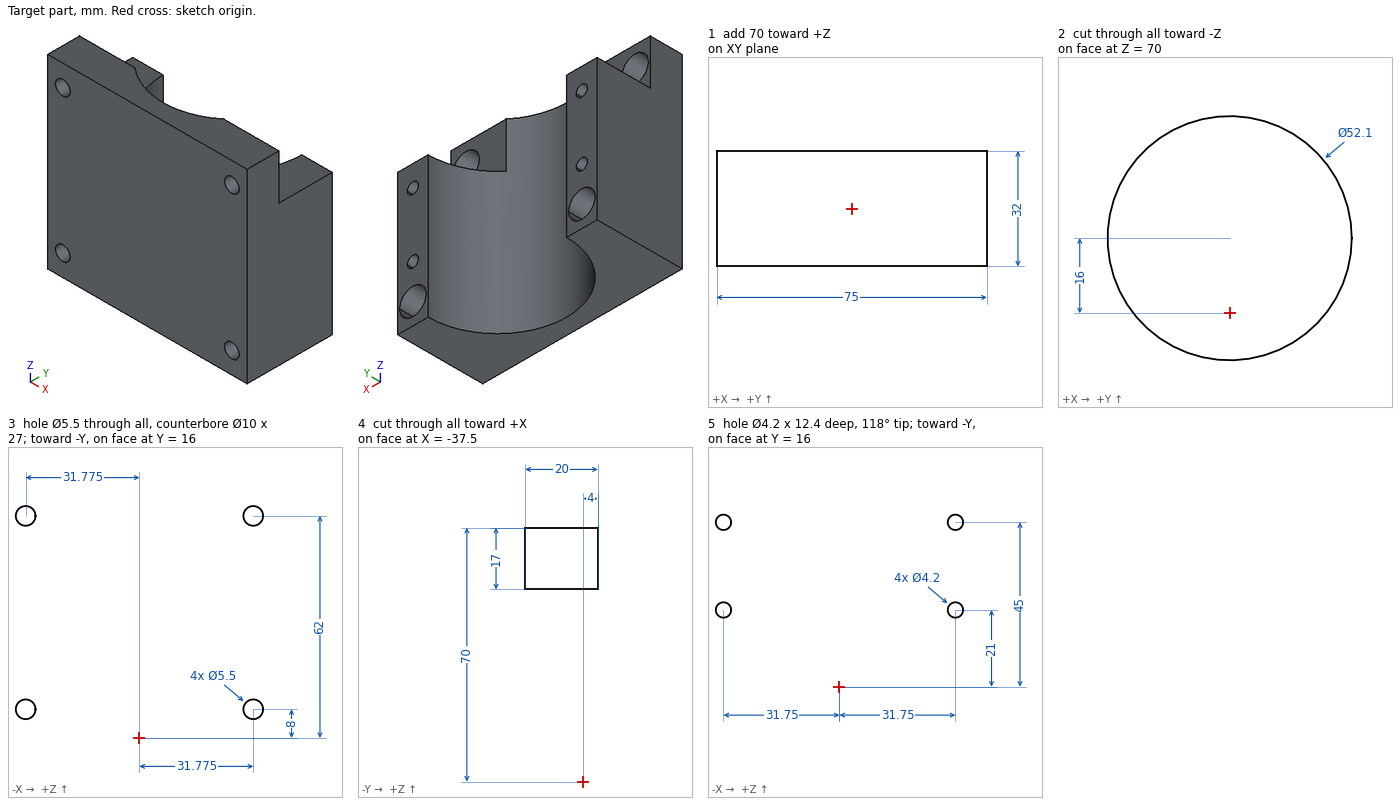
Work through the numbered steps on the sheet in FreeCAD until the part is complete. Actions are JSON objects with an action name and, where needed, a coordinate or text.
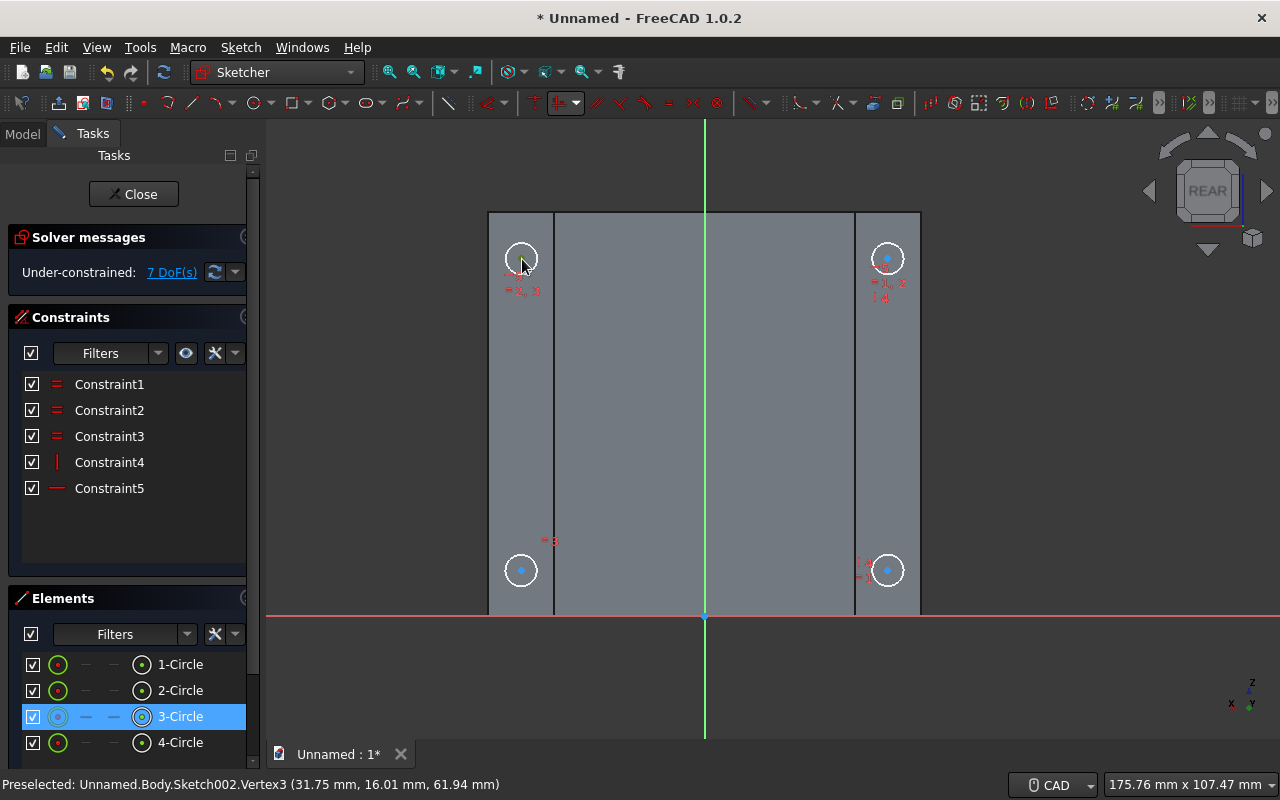
{"action": "left_click", "coordinate": [521, 571]}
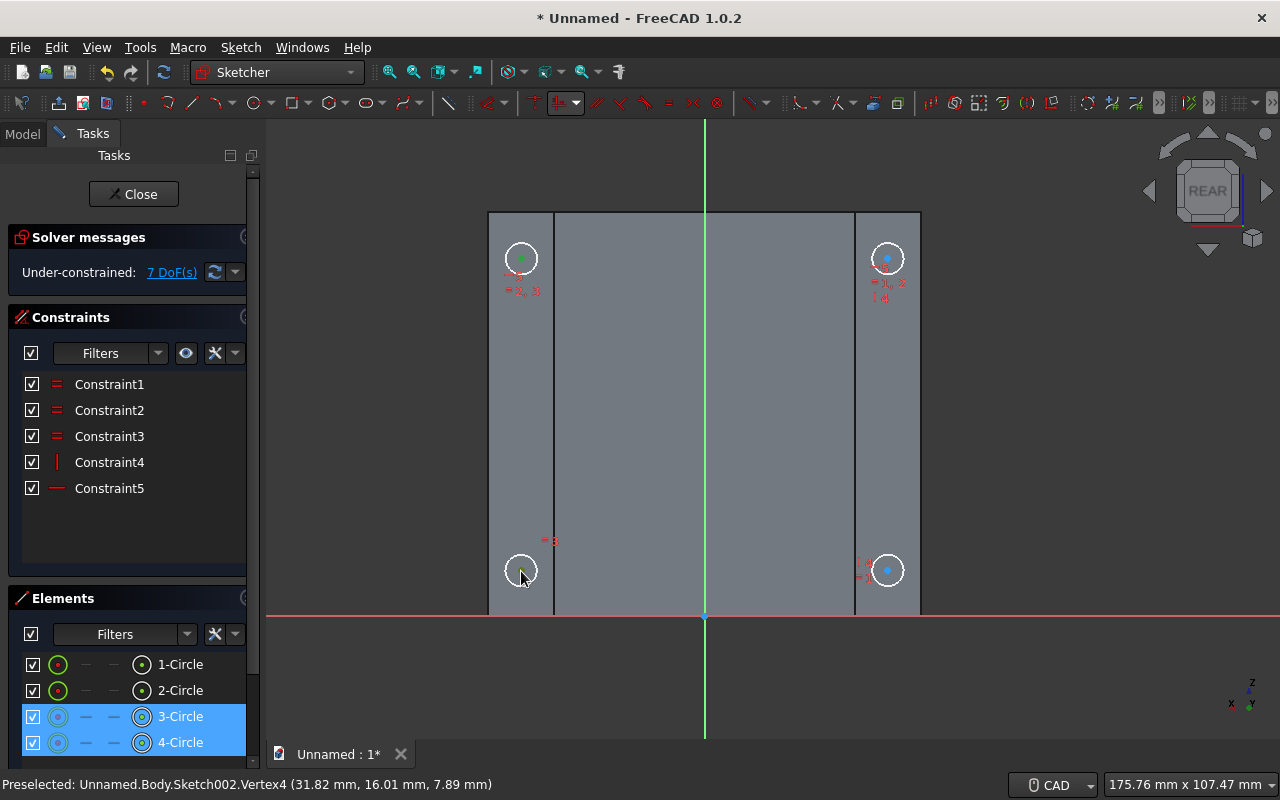
{"action": "key", "text": "v"}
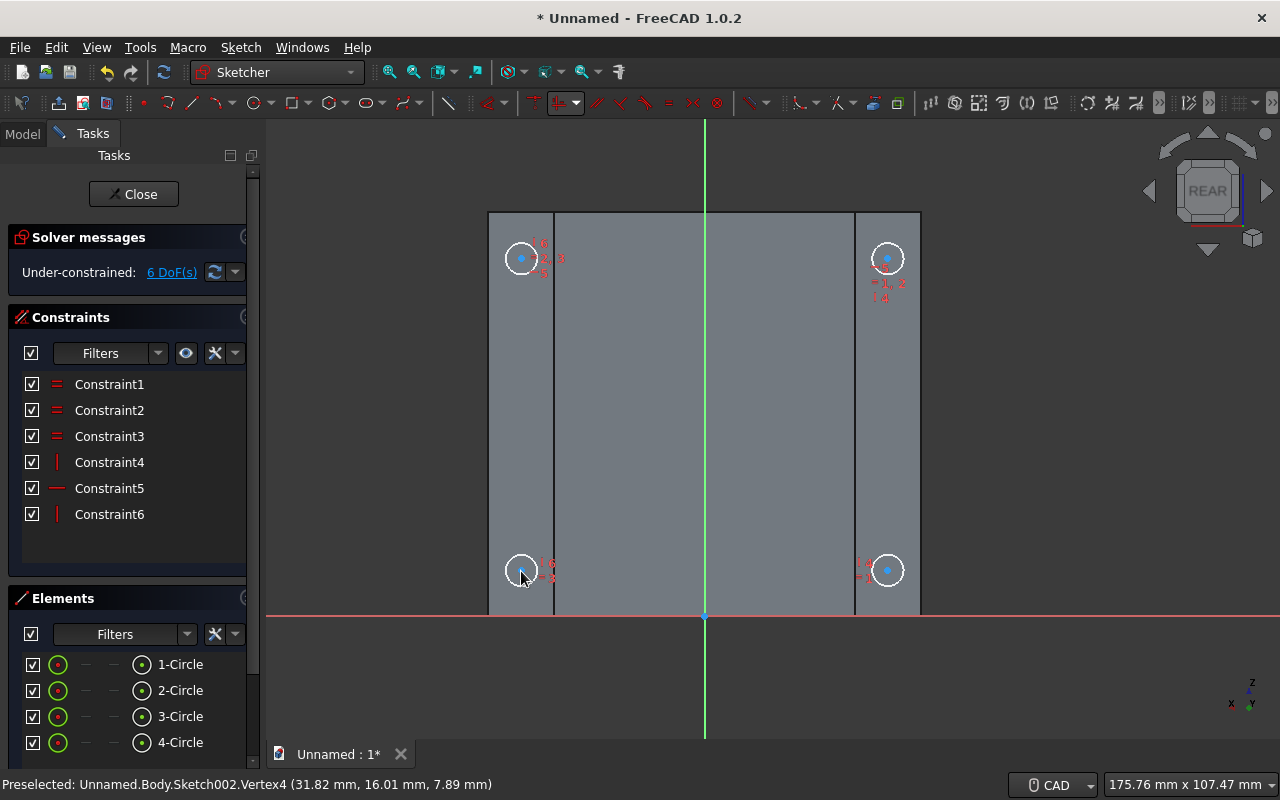
{"action": "left_click", "coordinate": [888, 570]}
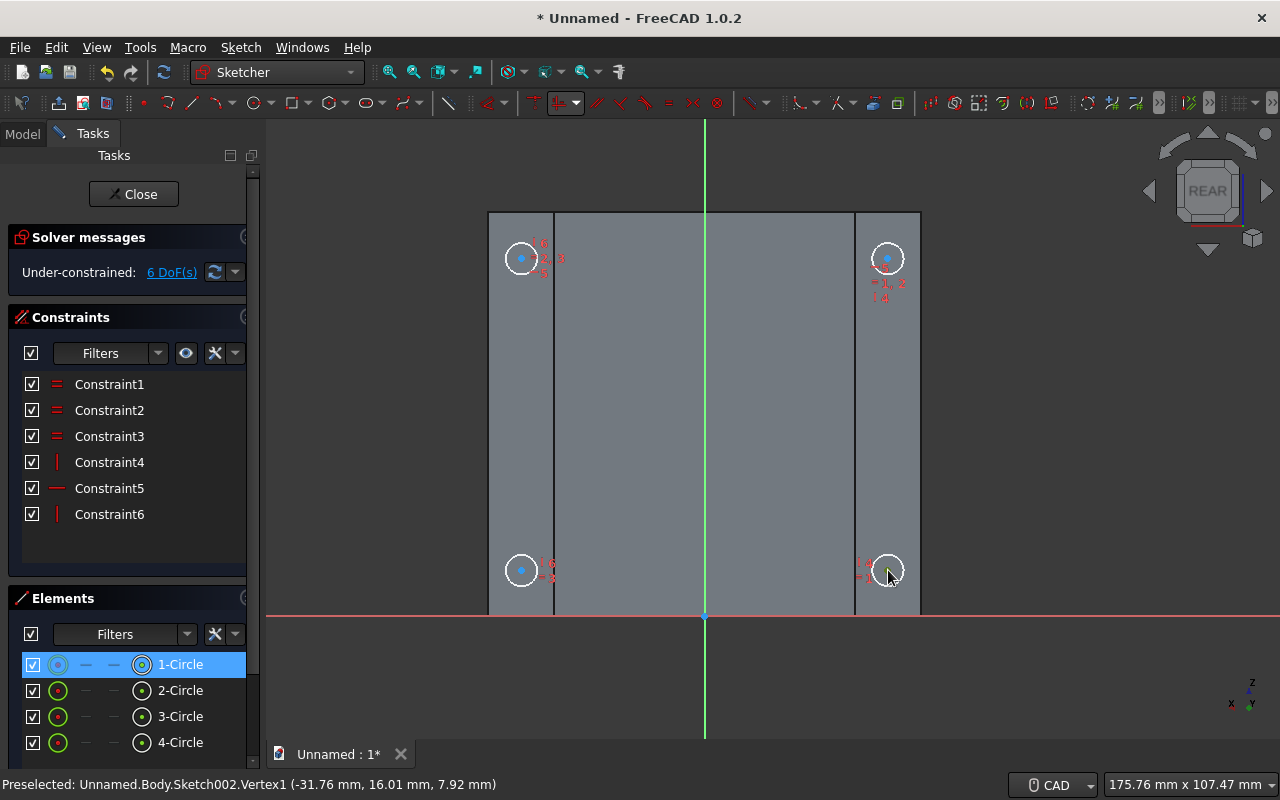
{"action": "left_click", "coordinate": [522, 571]}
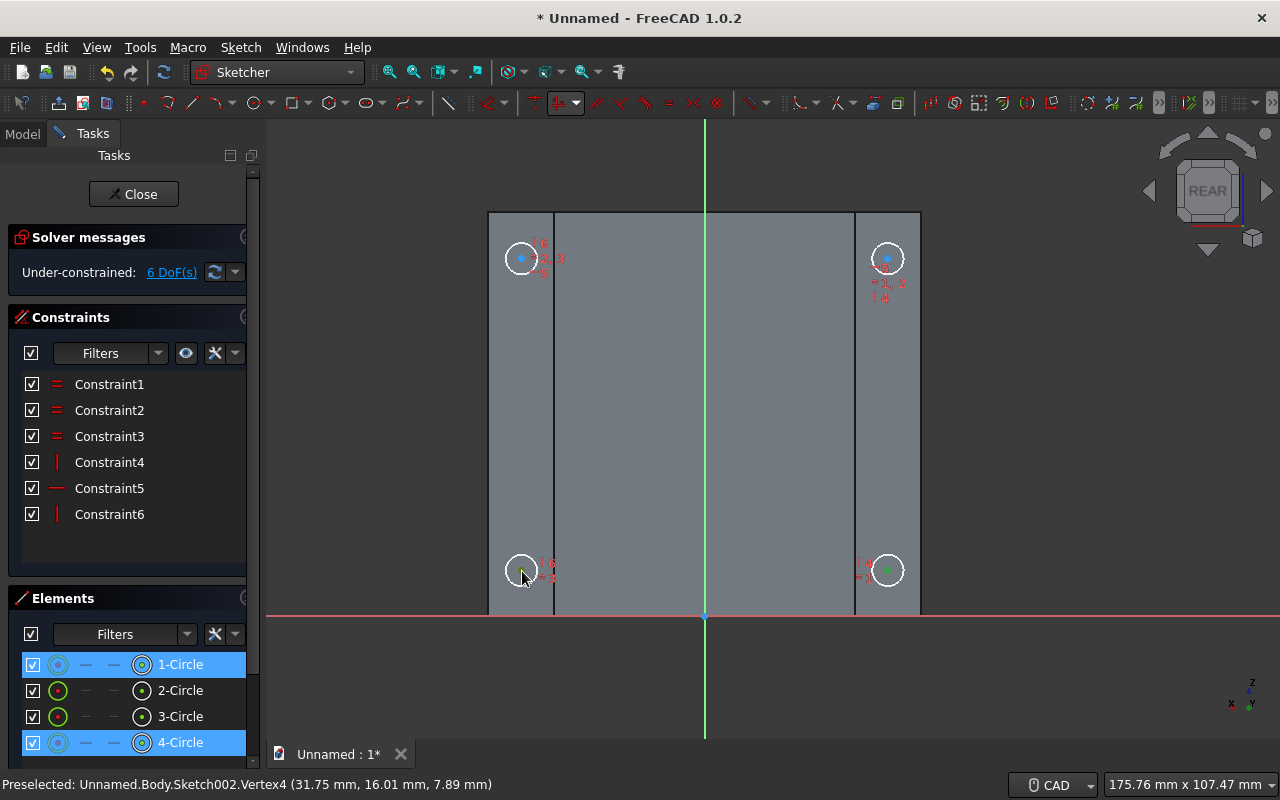
{"action": "key", "text": "h"}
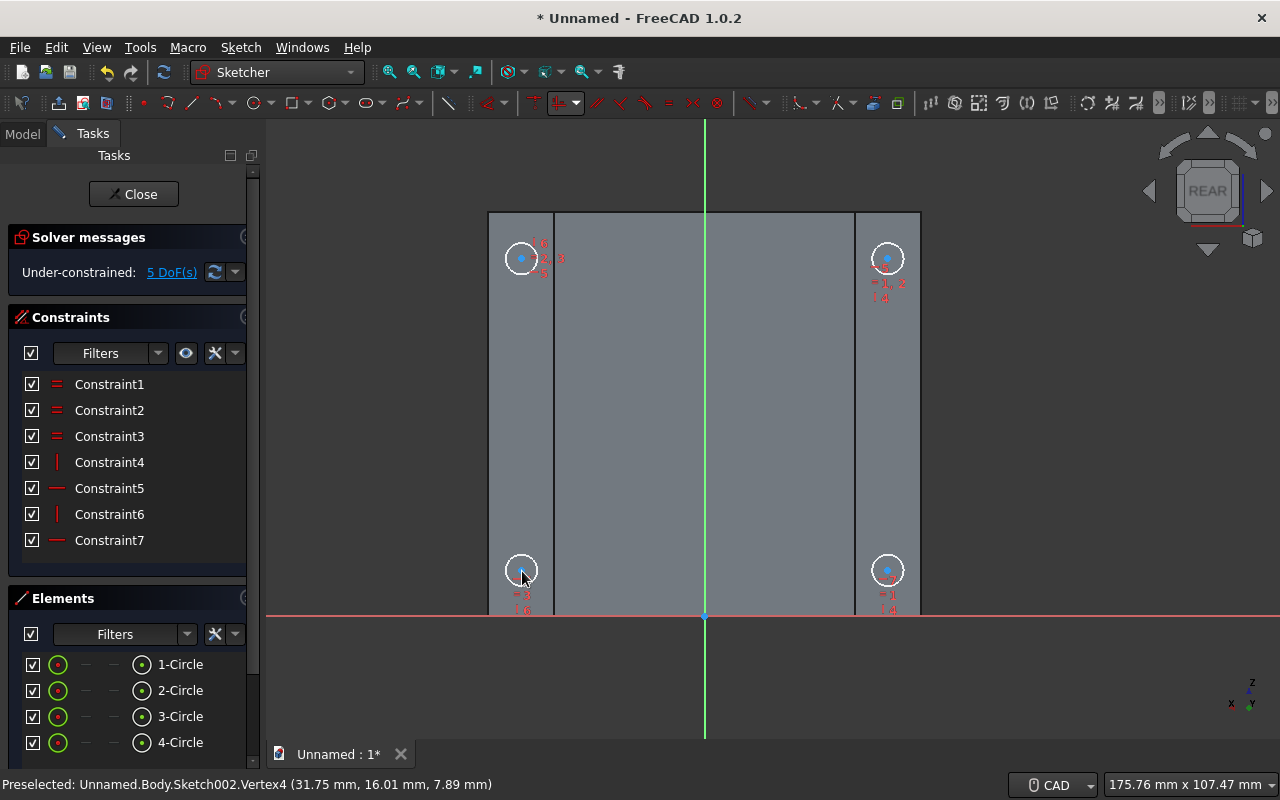
{"action": "left_click", "coordinate": [488, 104]}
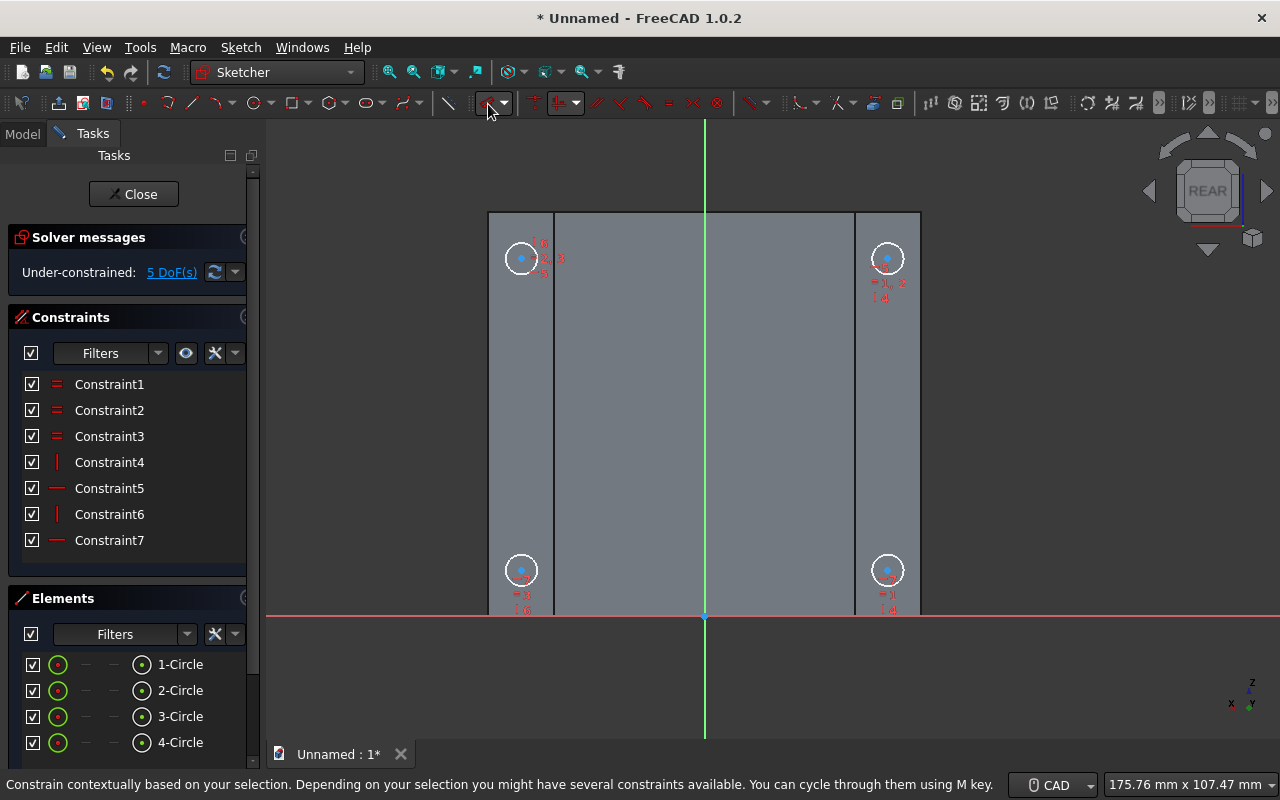
{"action": "scroll", "coordinate": [899, 559], "scroll_direction": "up", "scroll_amount": 2}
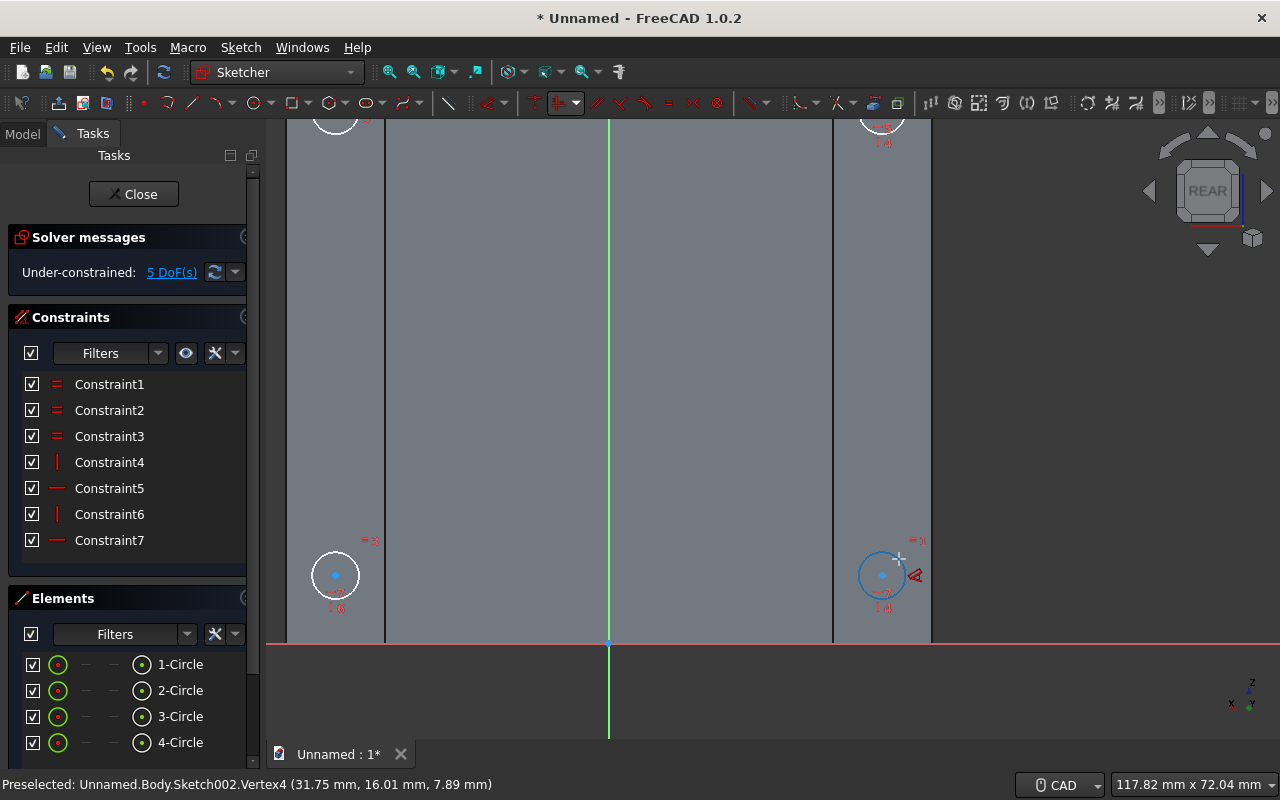
{"action": "left_click", "coordinate": [899, 559]}
{"action": "left_click", "coordinate": [922, 537]}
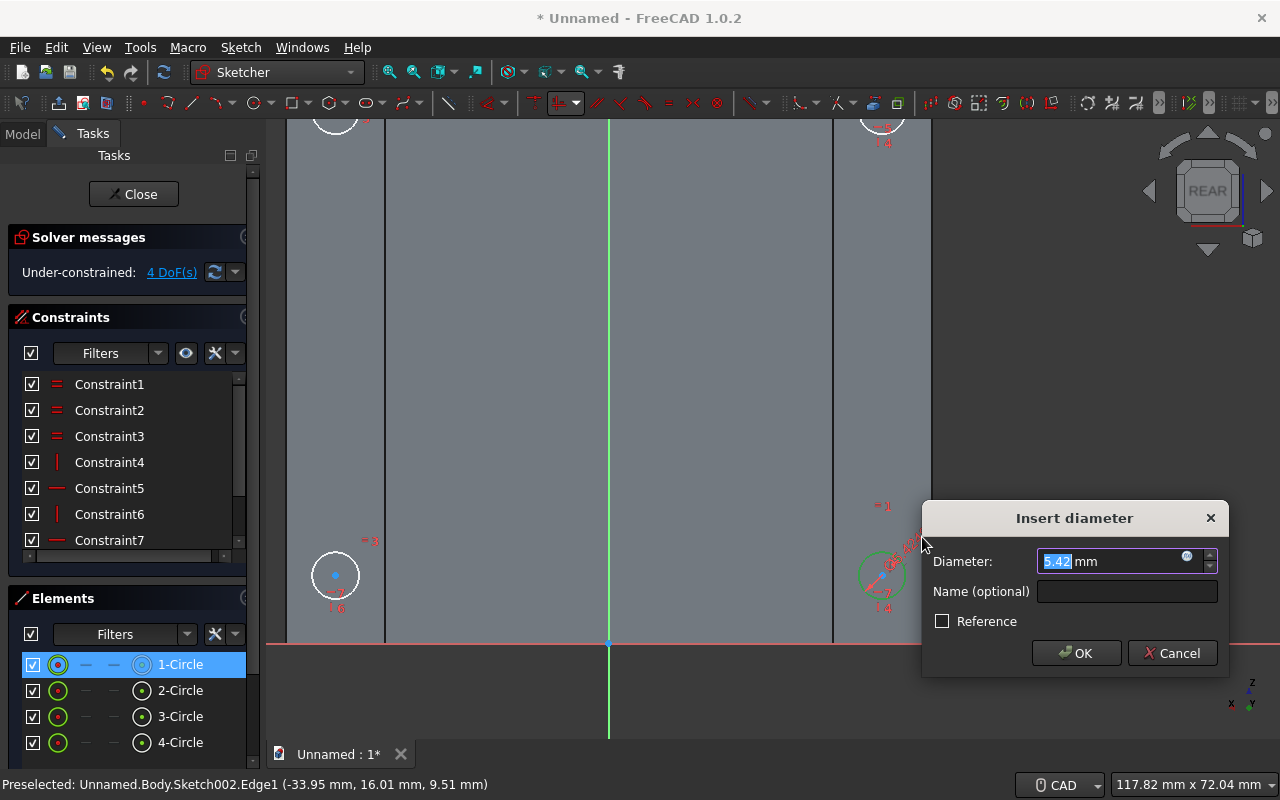
{"action": "type", "text": "5.5"}
{"action": "key", "text": "Return"}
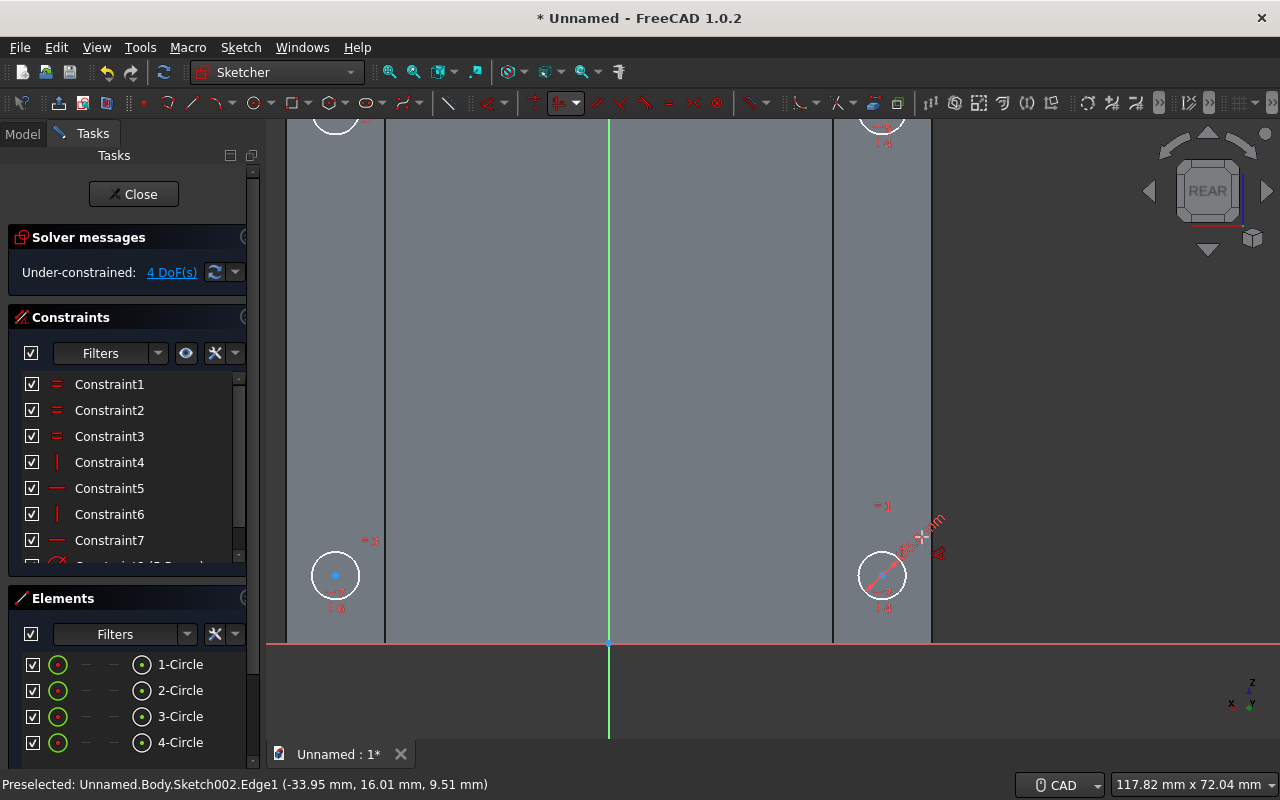
{"action": "left_click", "coordinate": [882, 576]}
{"action": "left_click", "coordinate": [916, 610]}